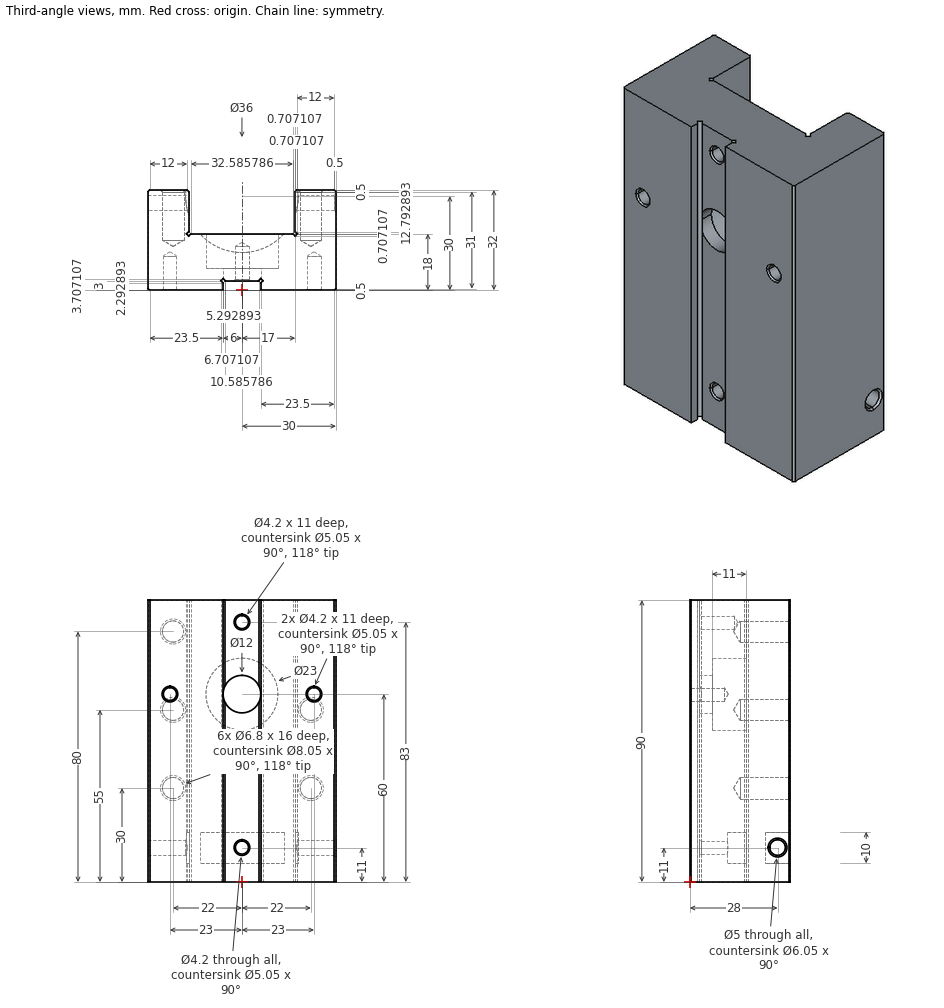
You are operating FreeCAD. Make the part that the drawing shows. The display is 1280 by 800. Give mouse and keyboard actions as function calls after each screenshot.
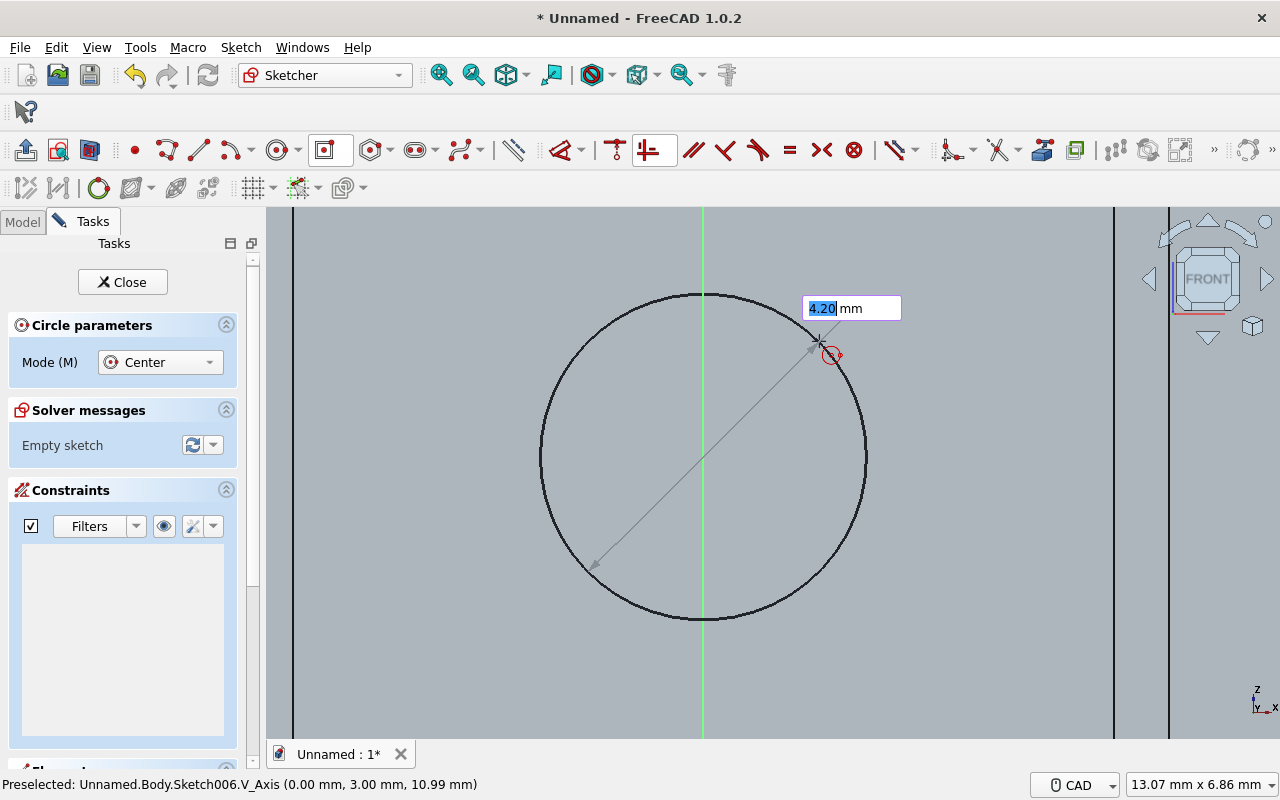
text(4.2)
key(Return)
key(Escape)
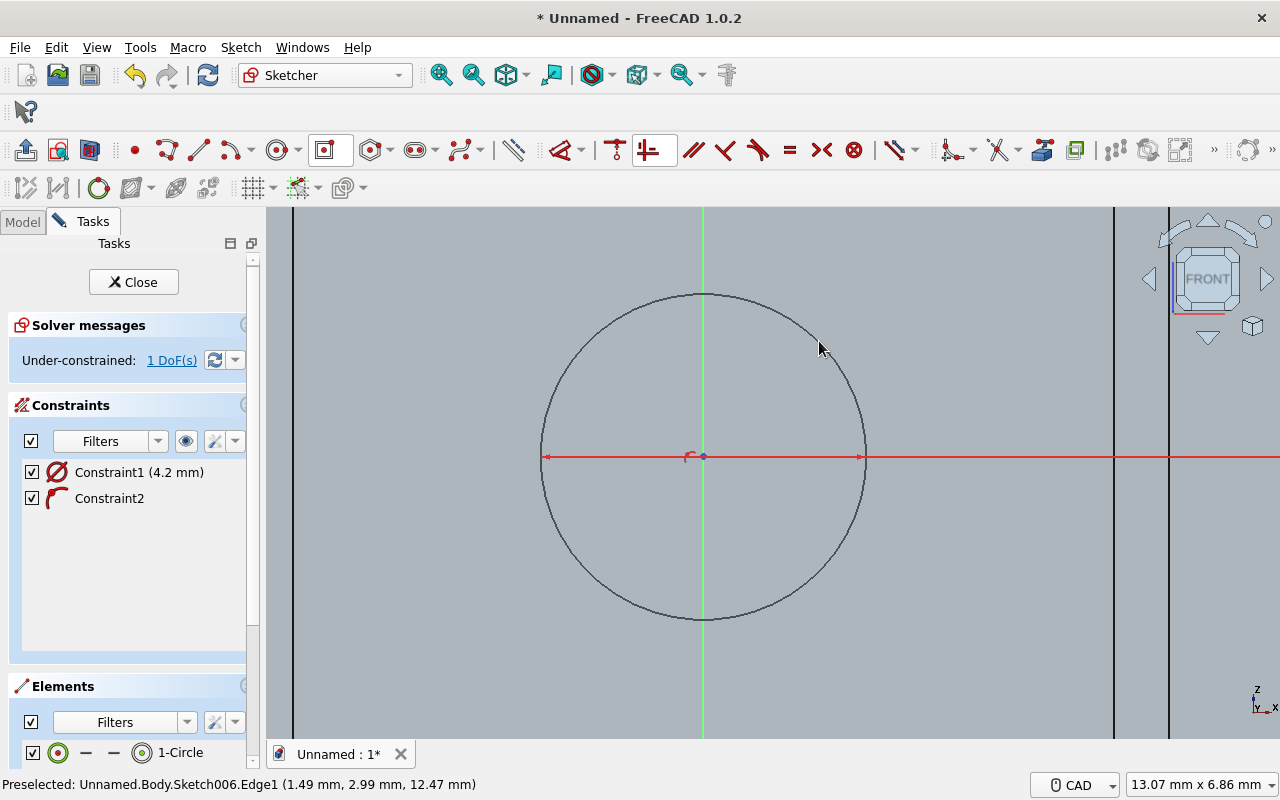
click(560, 150)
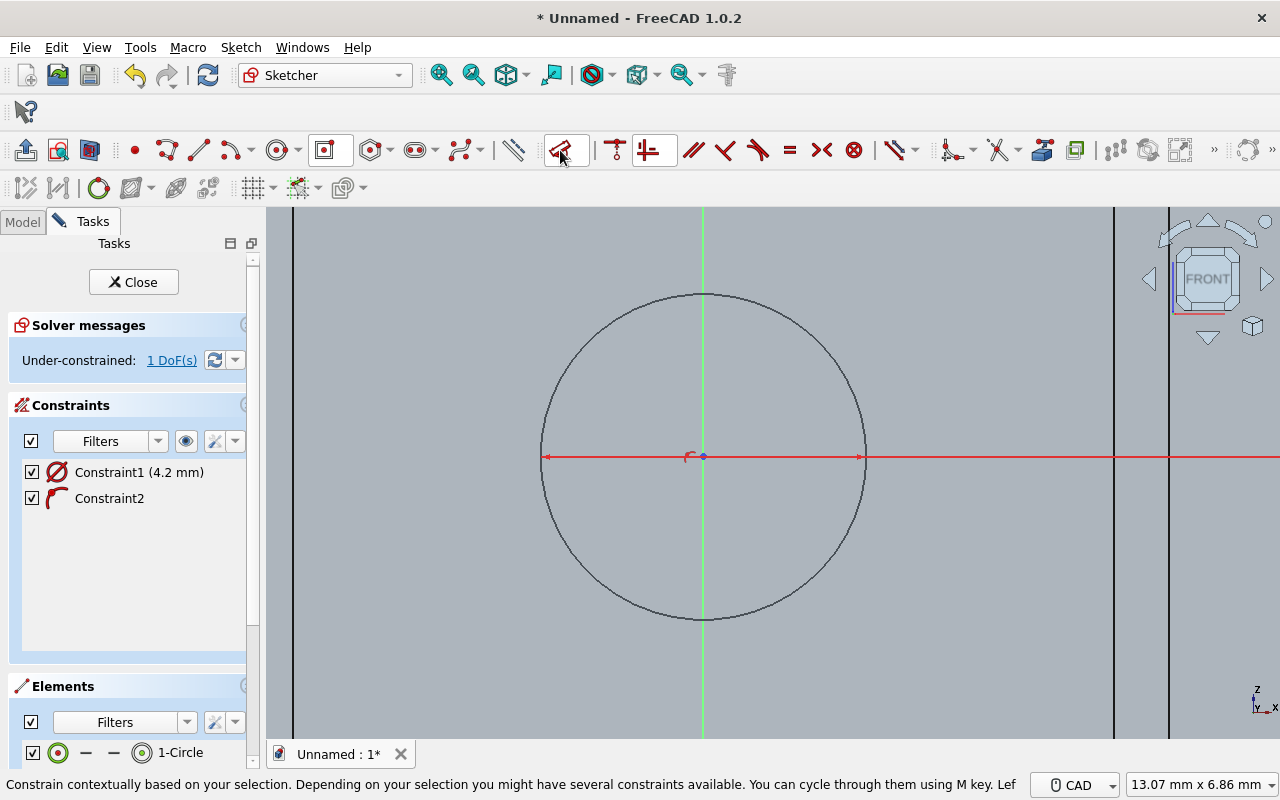
click(703, 457)
click(737, 584)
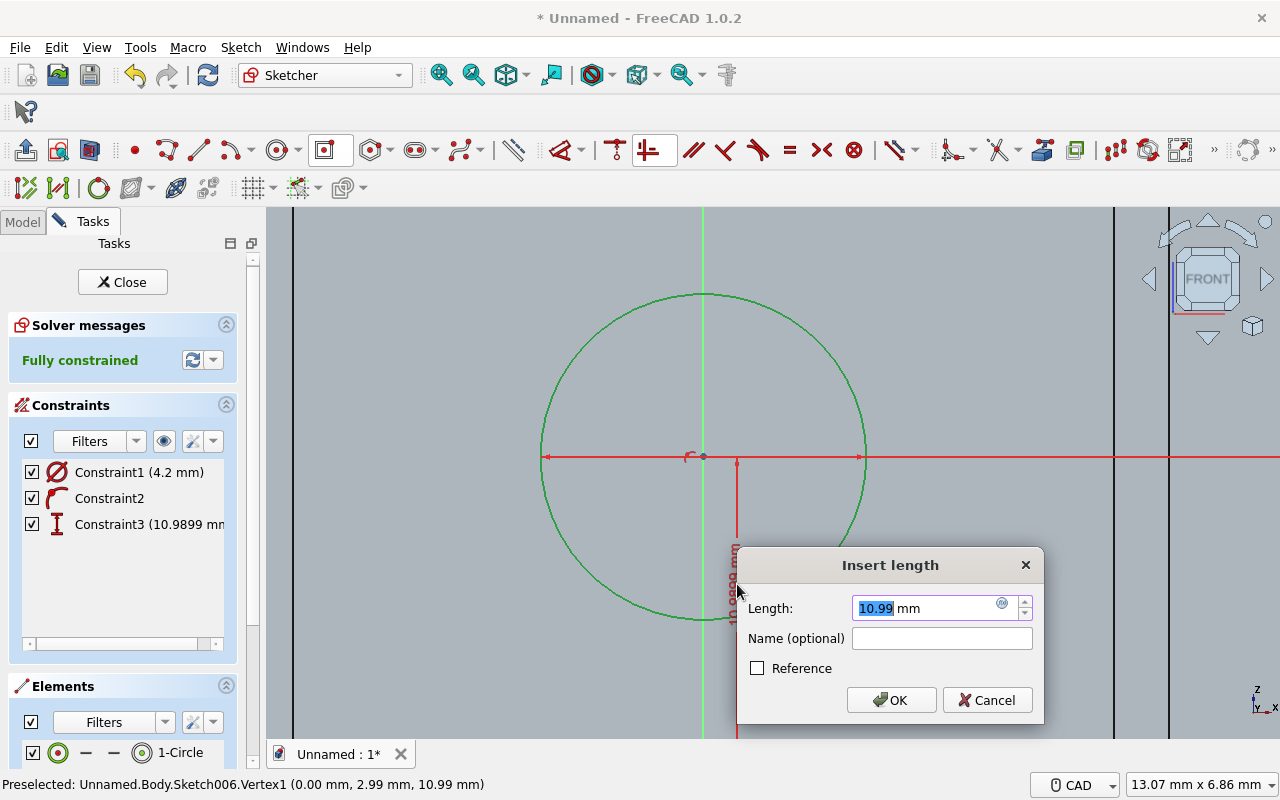
text(11)
key(Return)
key(Escape)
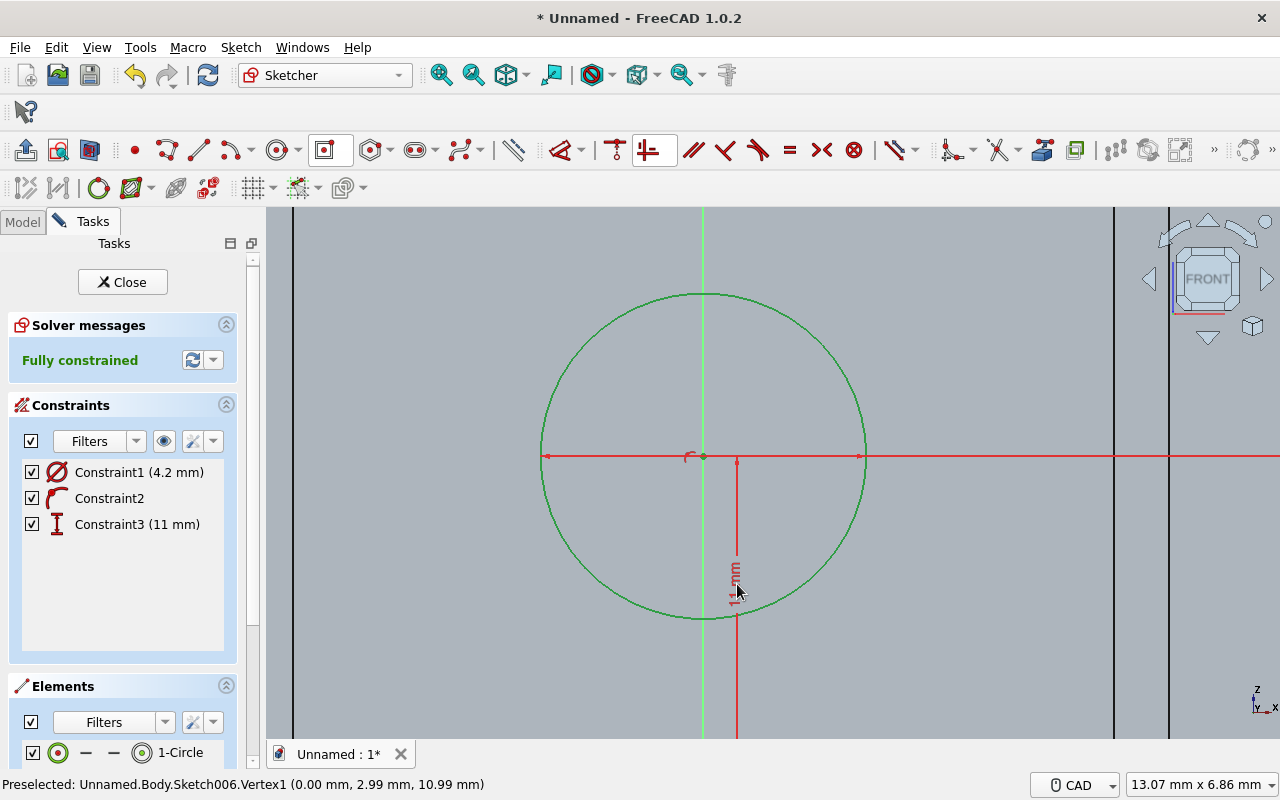
click(123, 282)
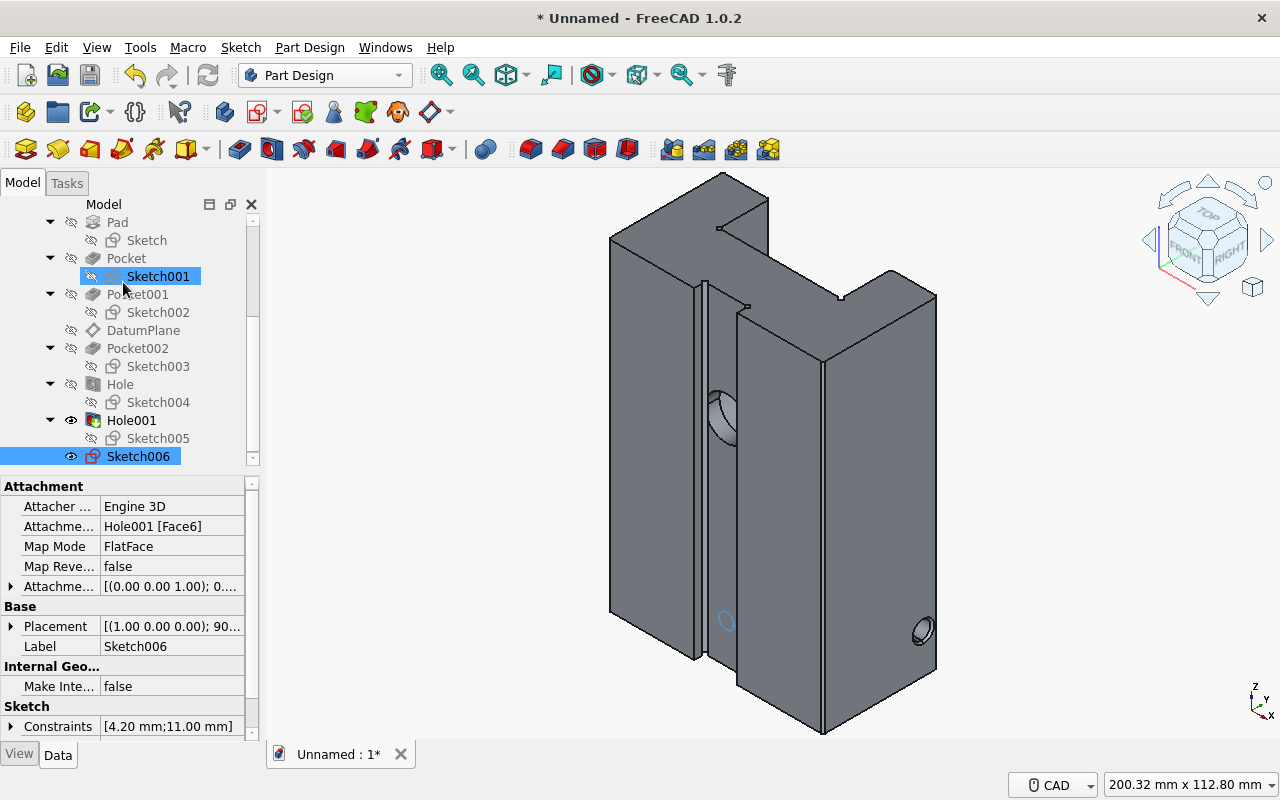
click(272, 150)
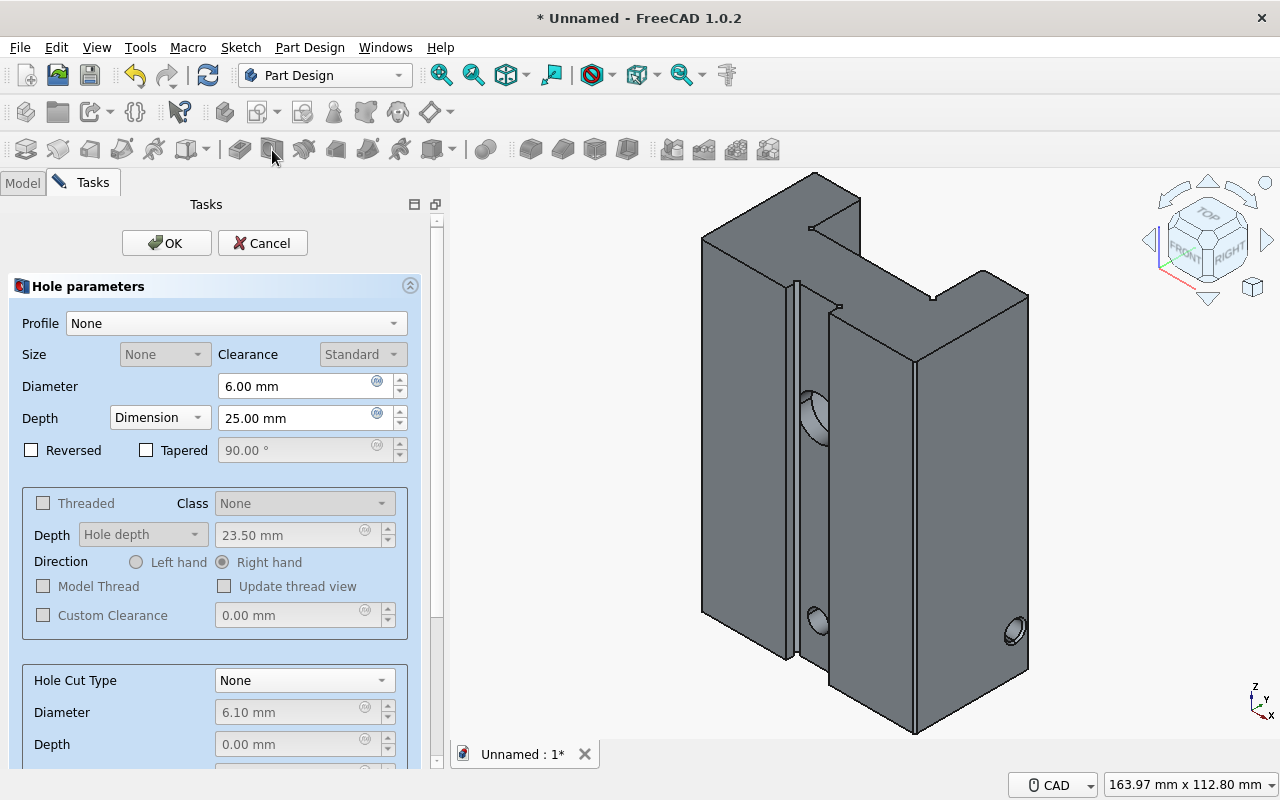
triple_click(305, 386)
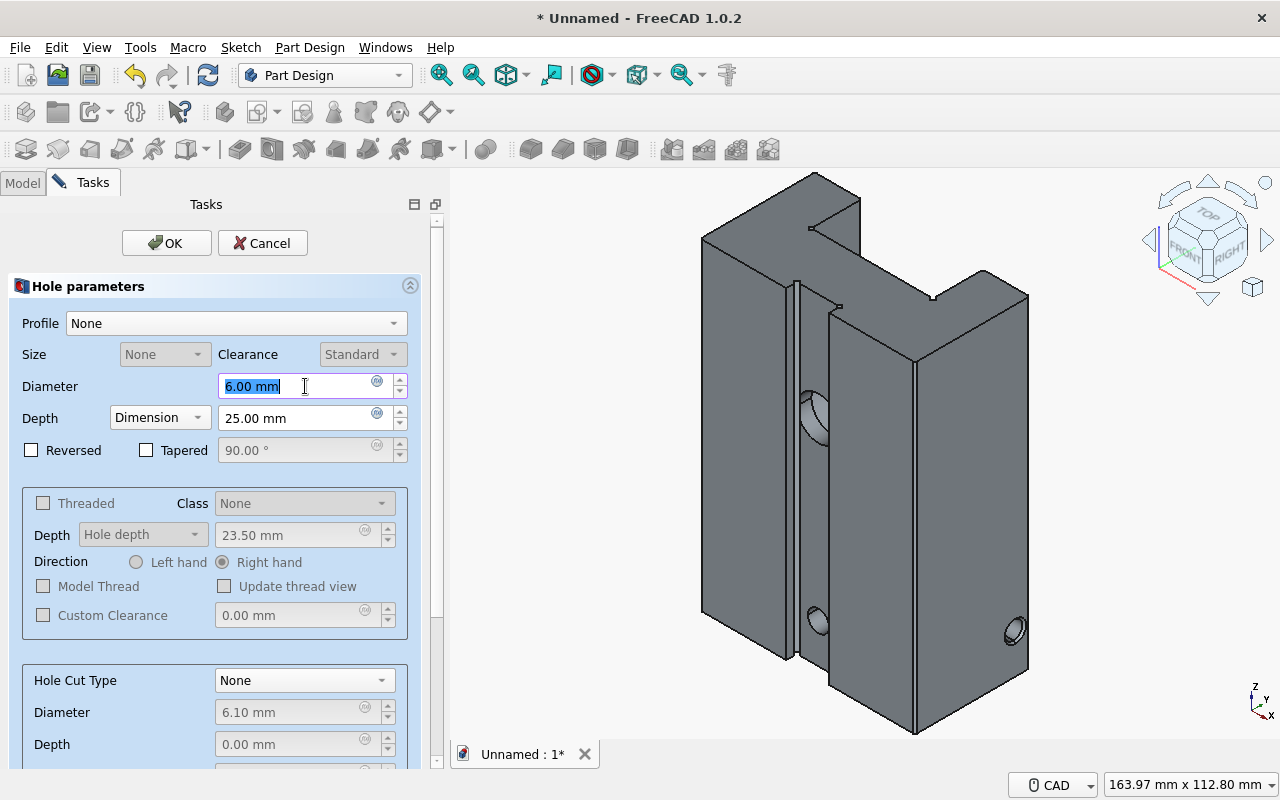
text(4.2)
key(Tab)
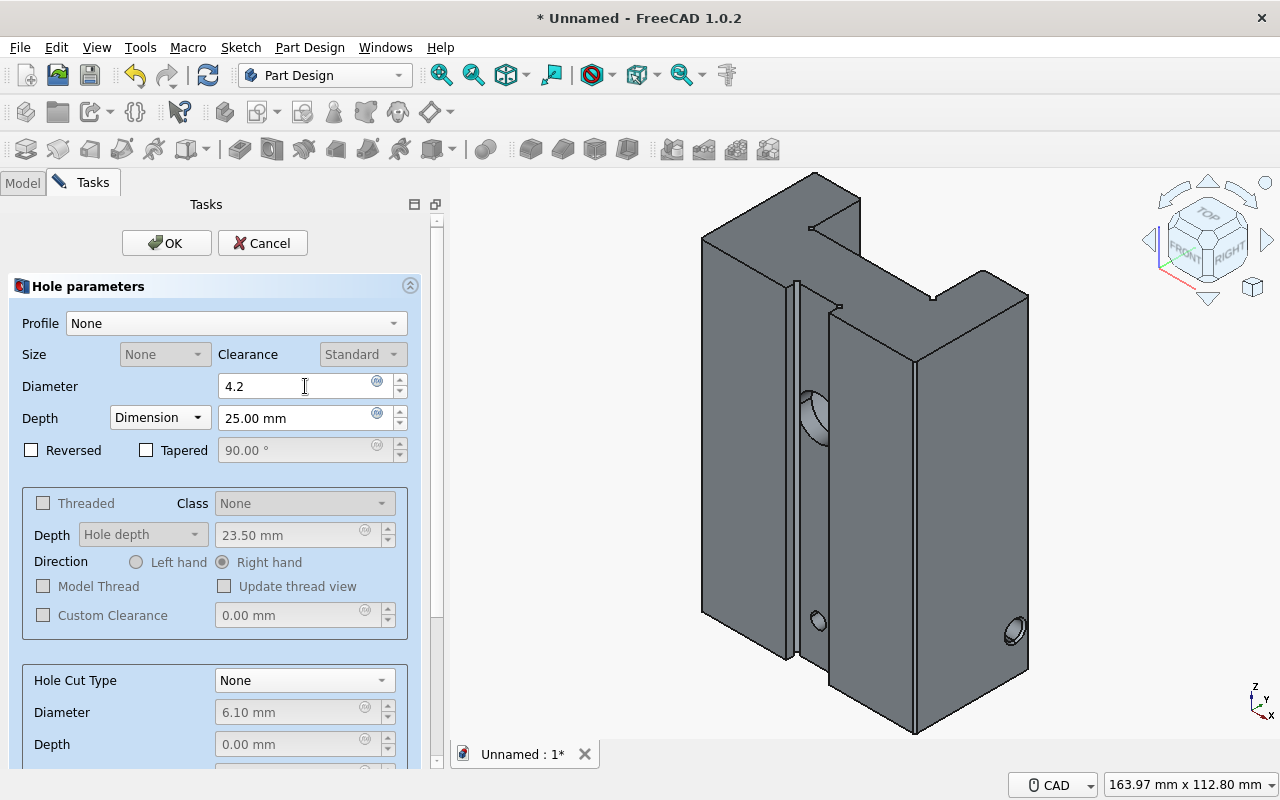
click(161, 418)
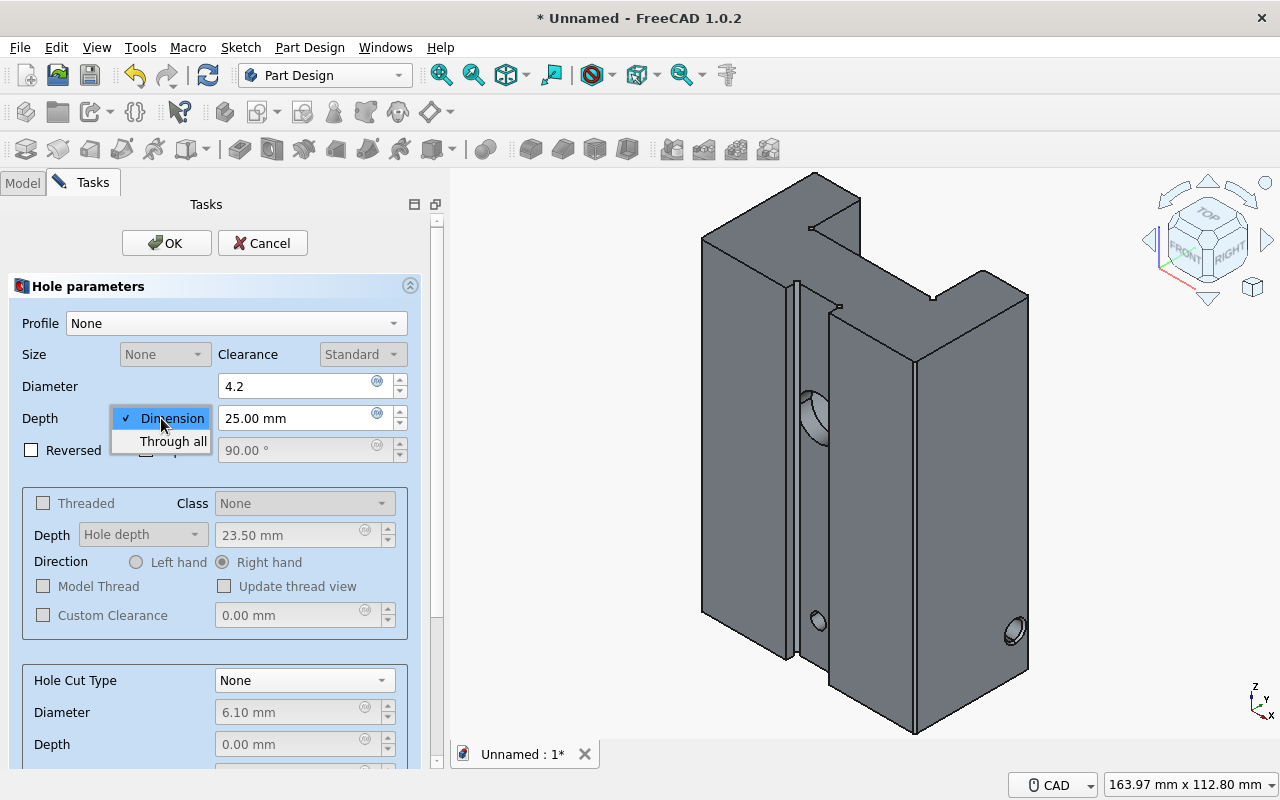
click(160, 442)